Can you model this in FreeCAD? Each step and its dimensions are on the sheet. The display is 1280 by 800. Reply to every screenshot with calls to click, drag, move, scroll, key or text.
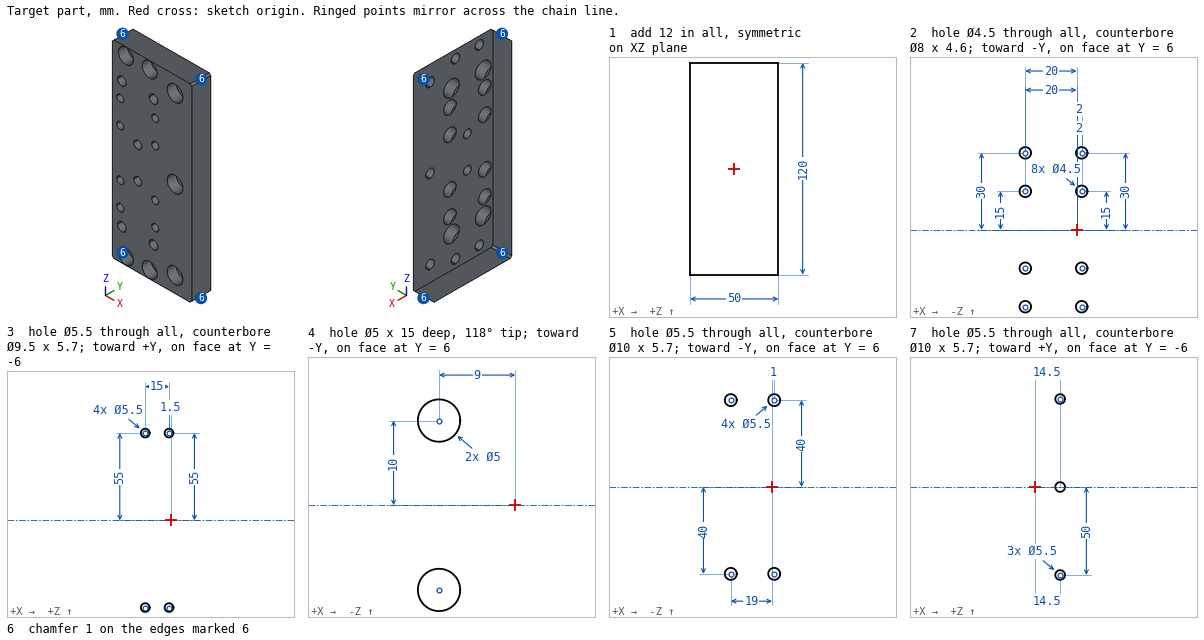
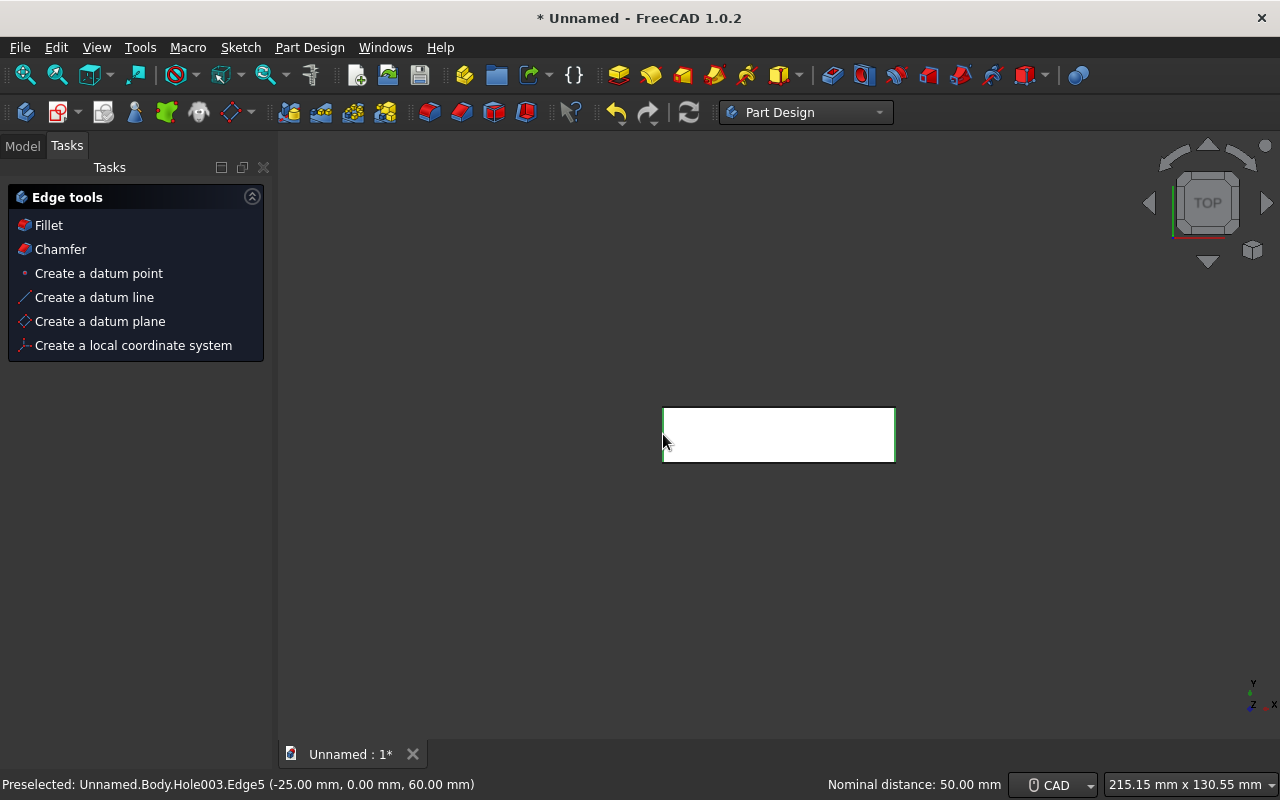
key(1)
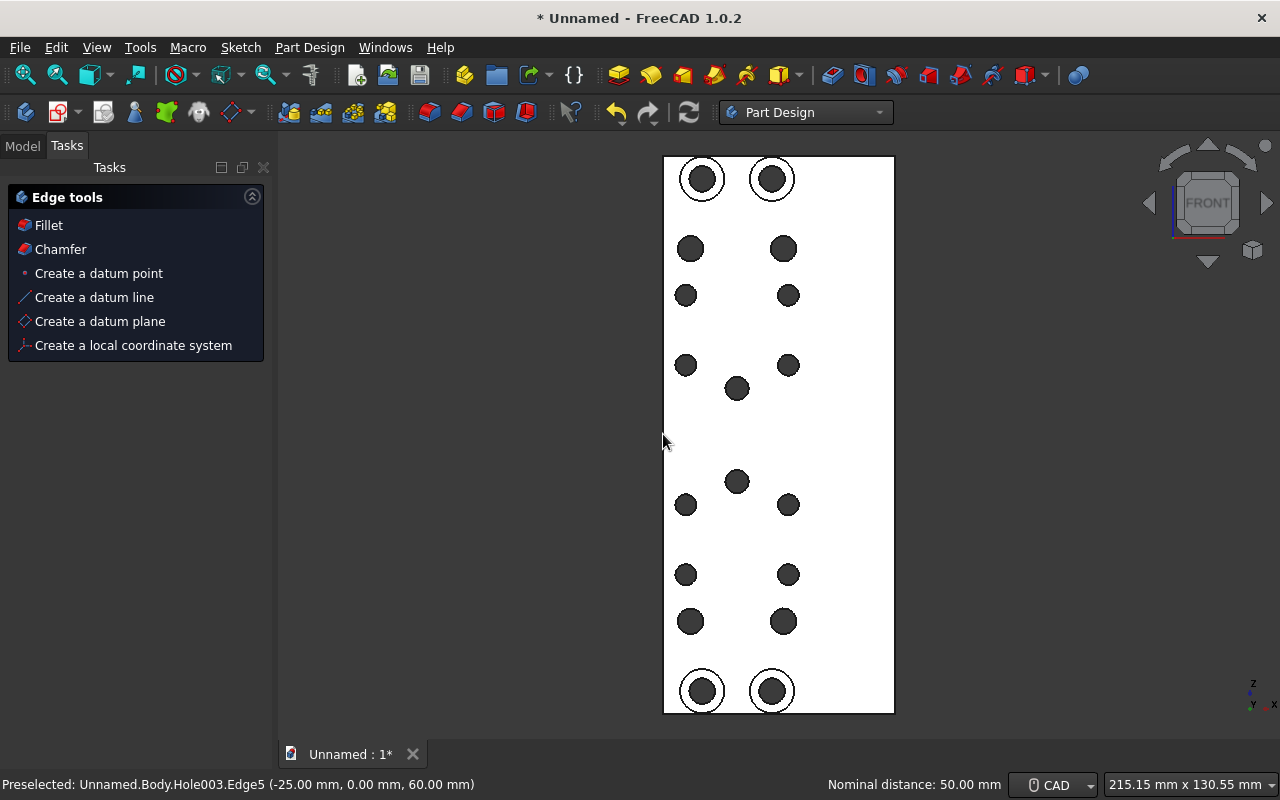
key(3)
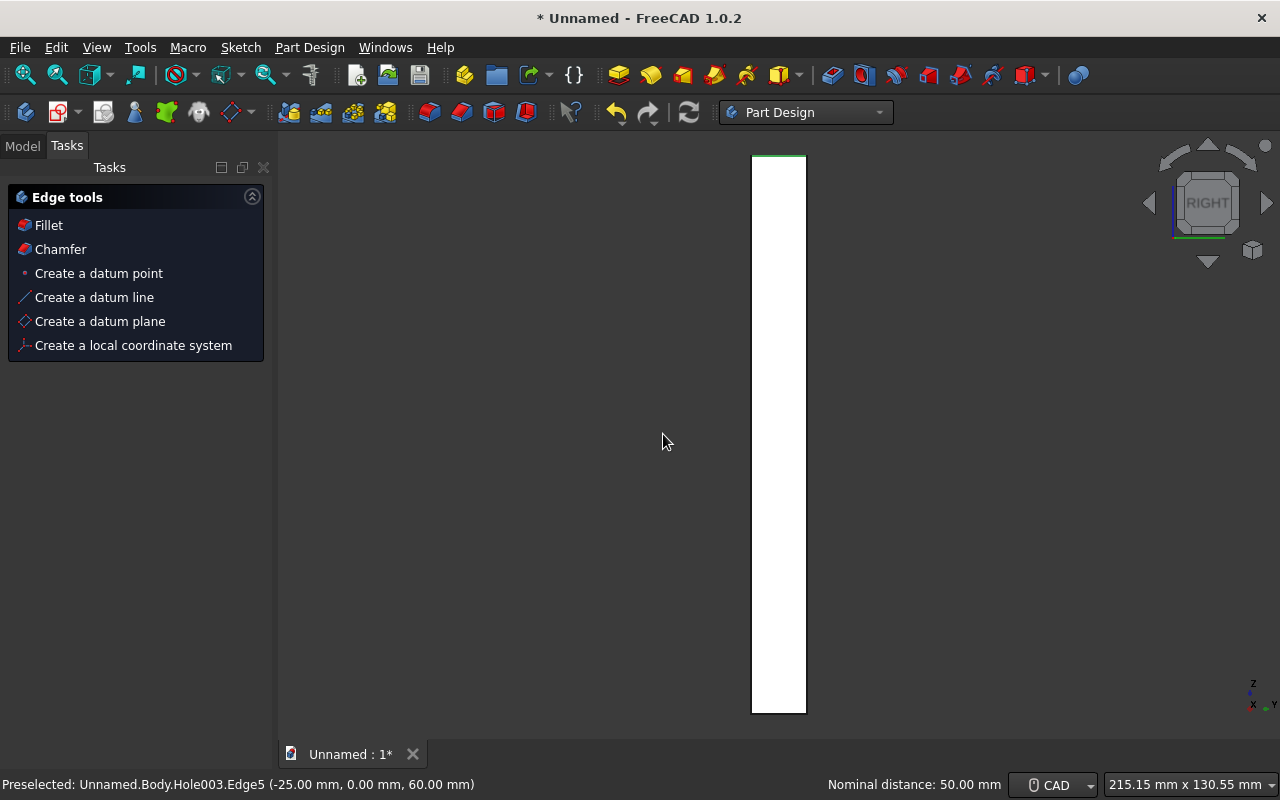
key(5)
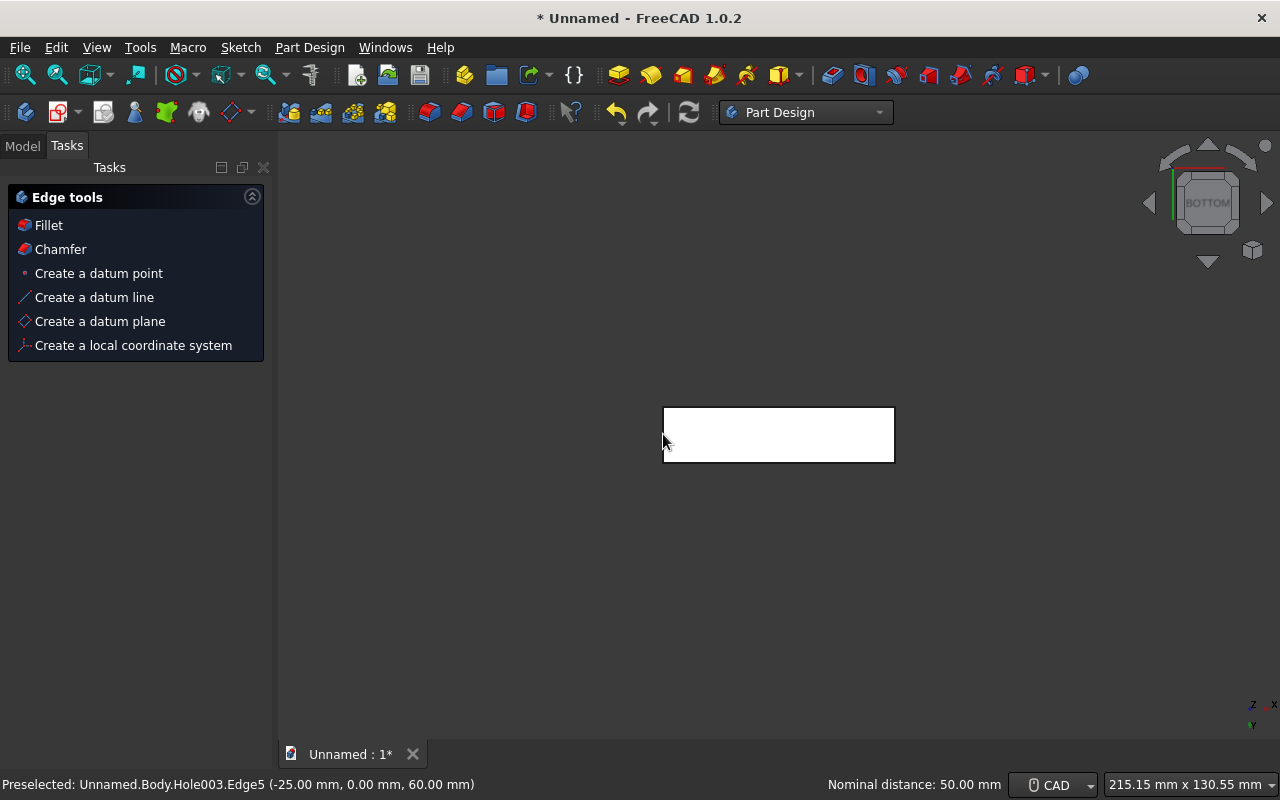
click(26, 76)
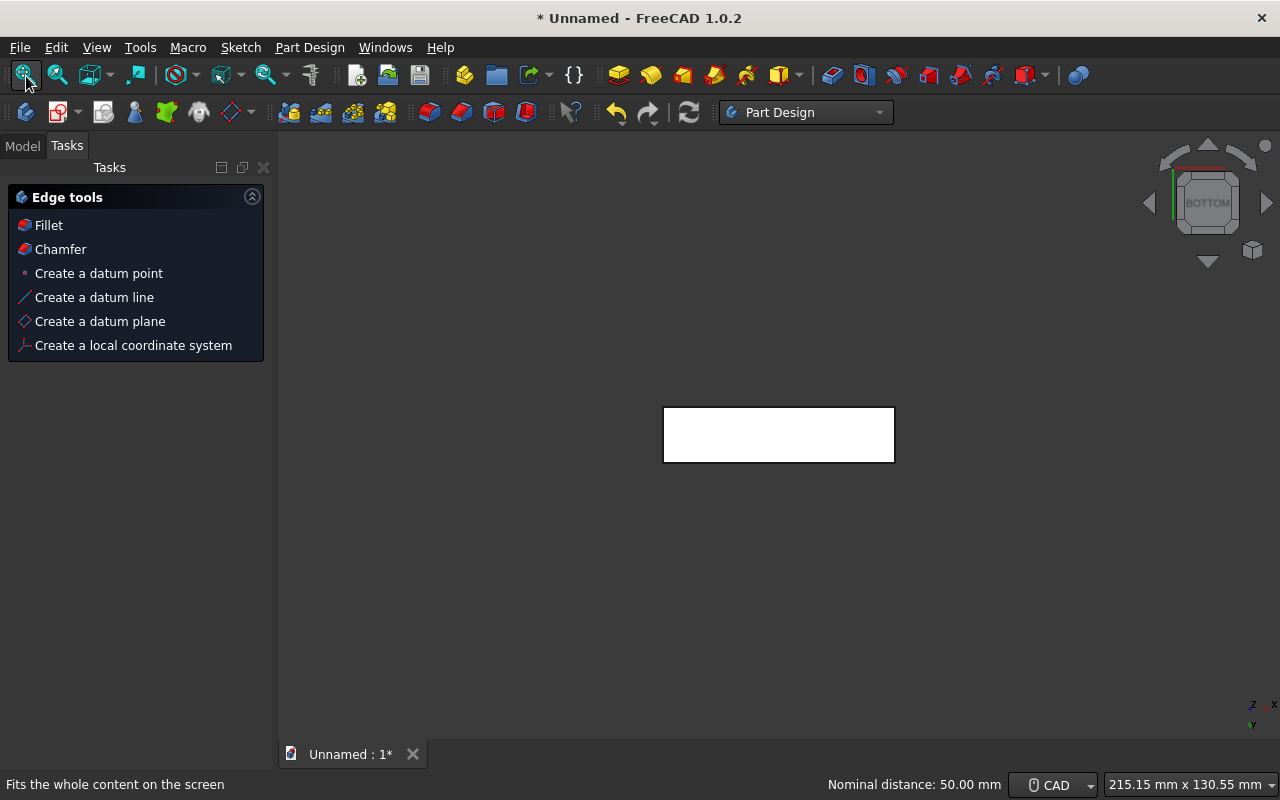
click(663, 434, ctrl)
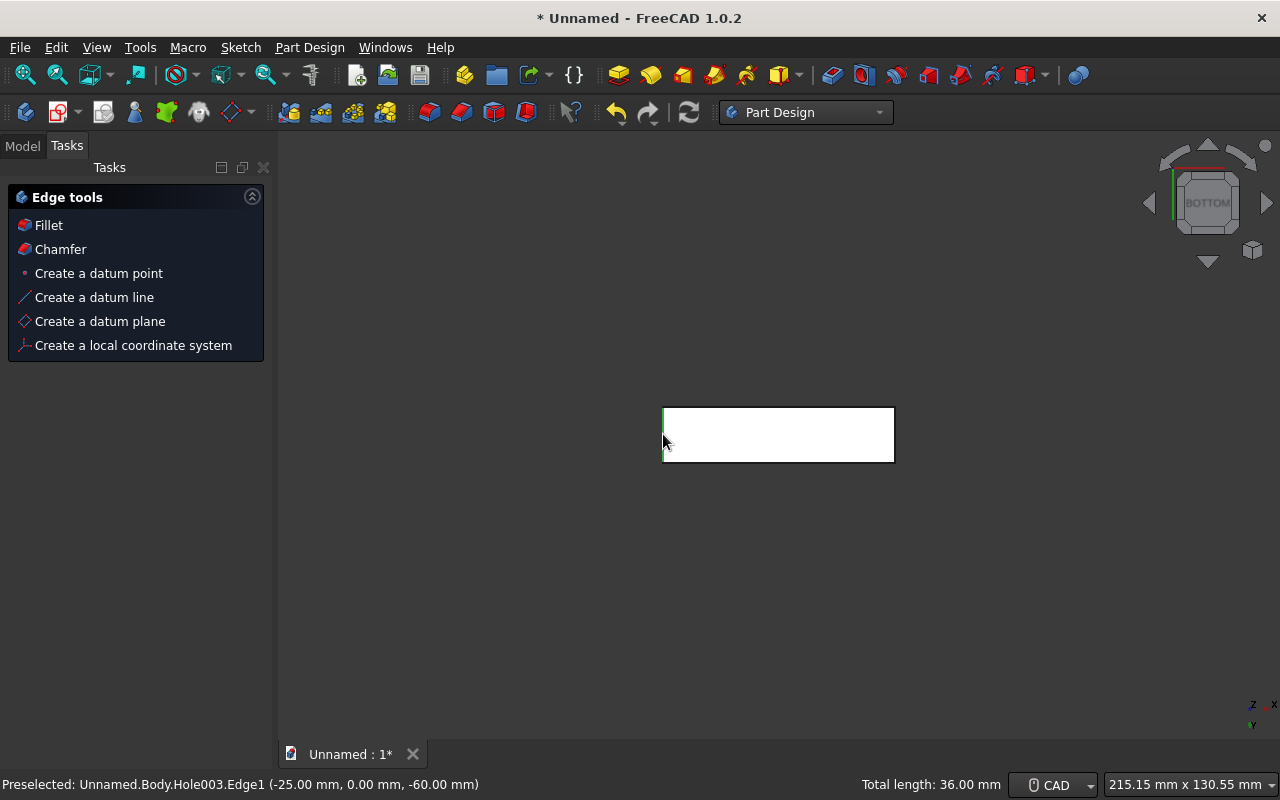
click(895, 434, ctrl)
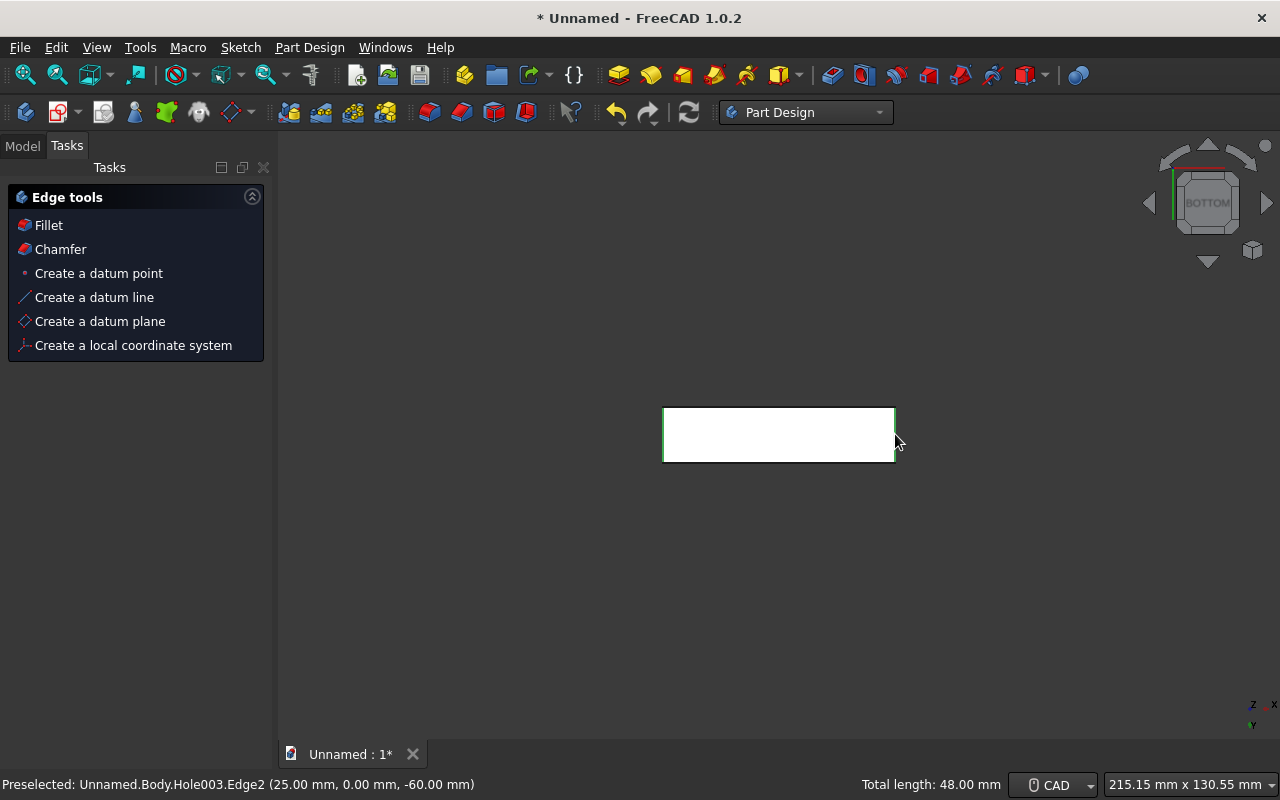
click(462, 112)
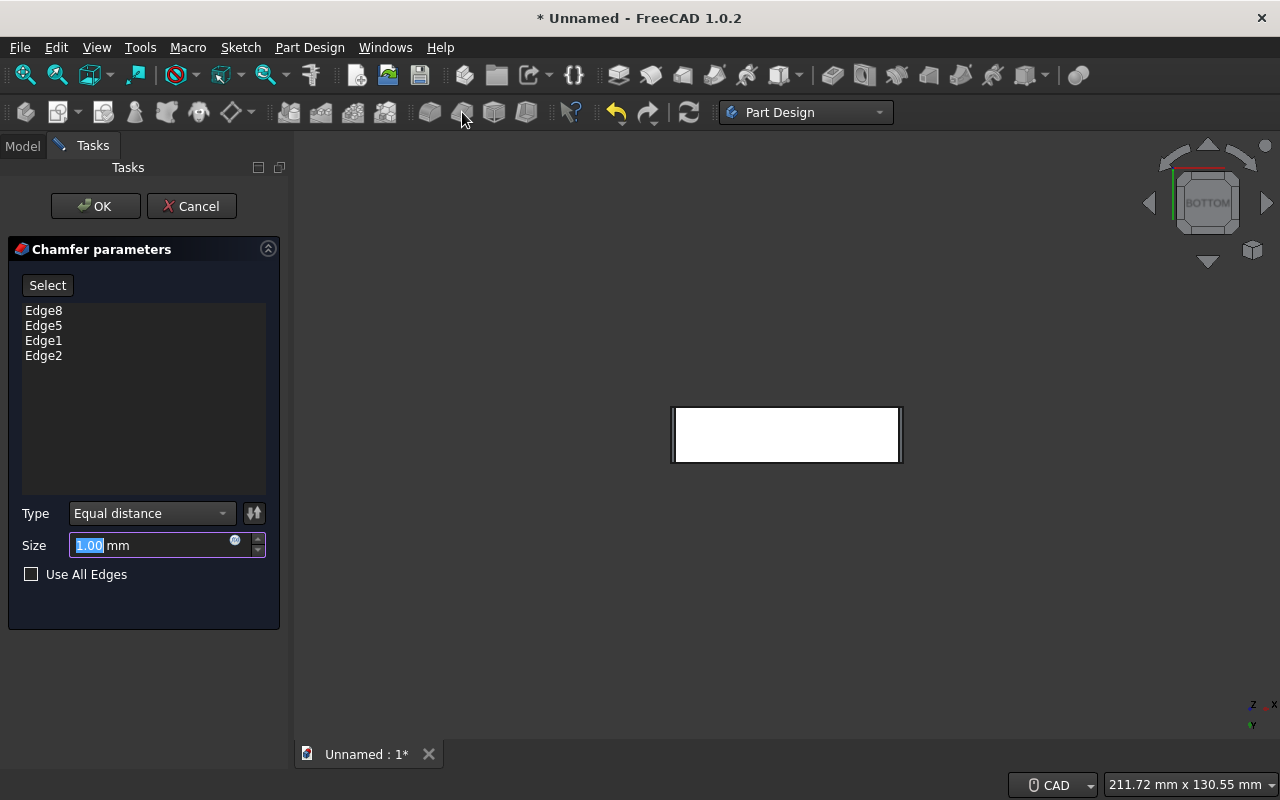
text(1)
key(Tab)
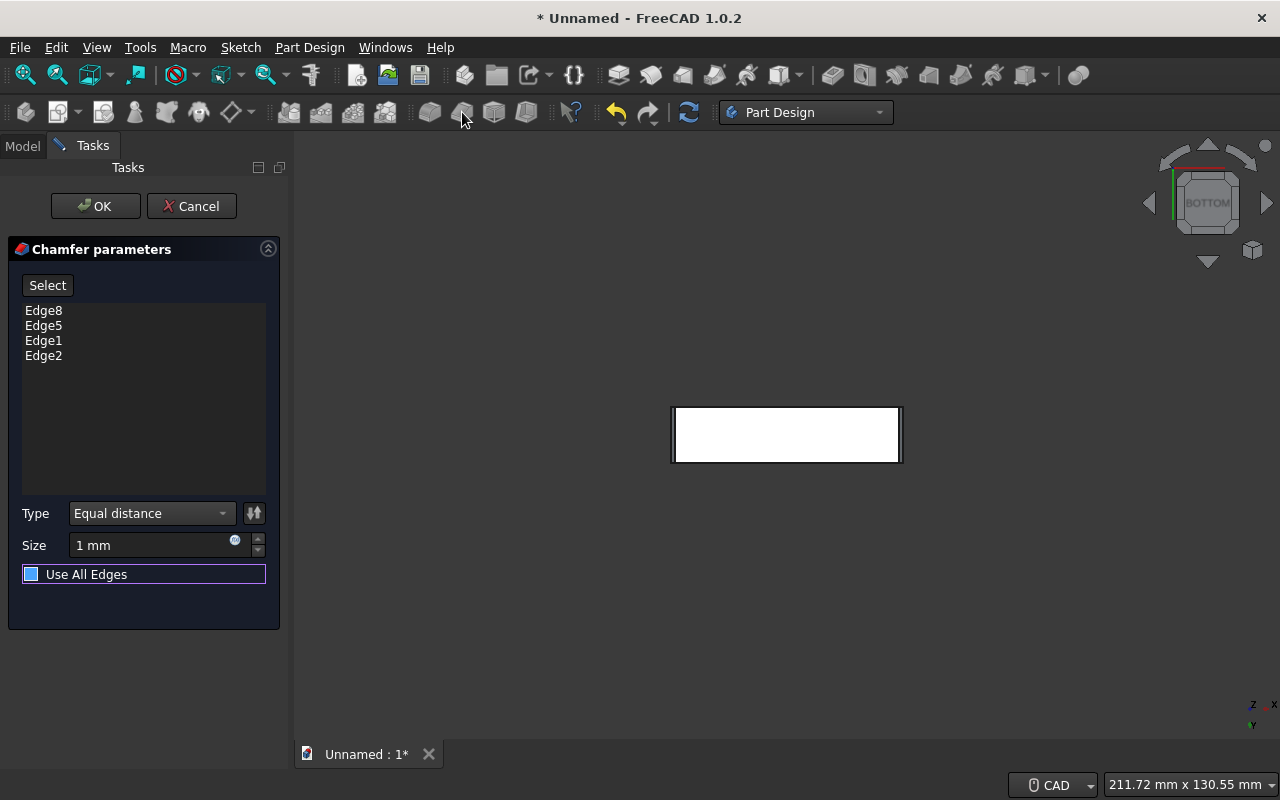
click(96, 206)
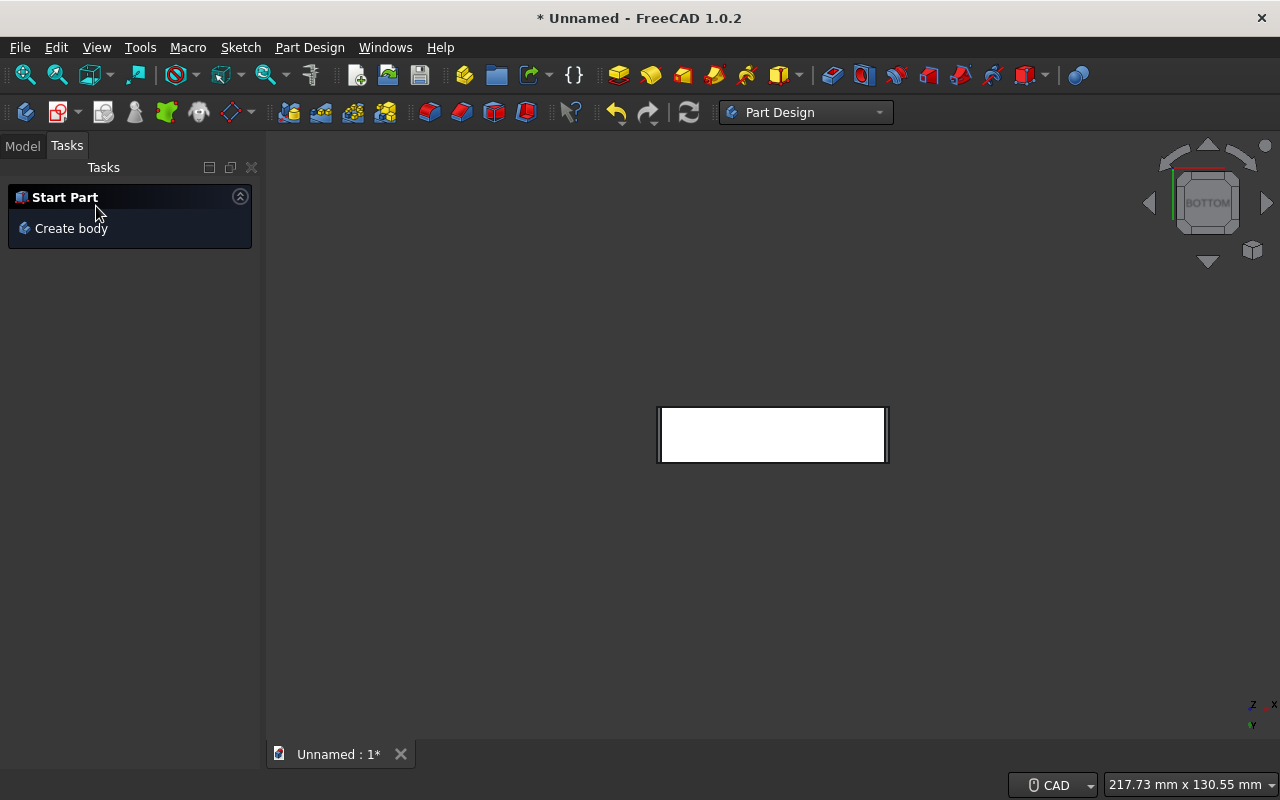
click(26, 76)